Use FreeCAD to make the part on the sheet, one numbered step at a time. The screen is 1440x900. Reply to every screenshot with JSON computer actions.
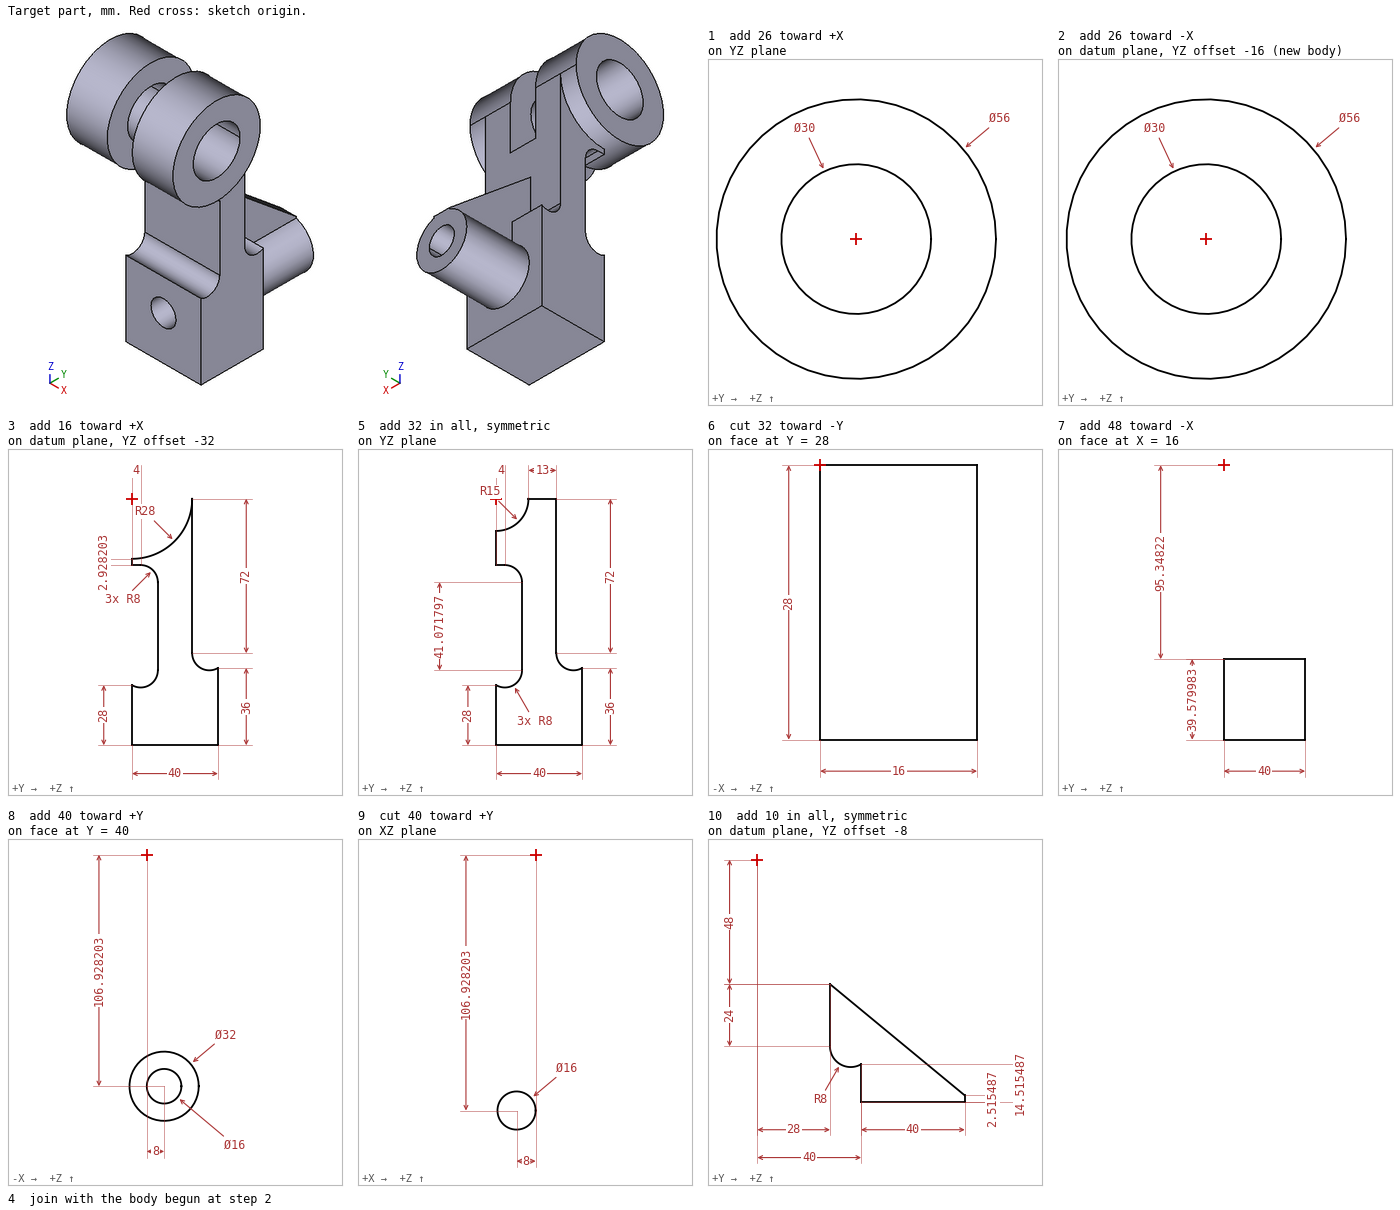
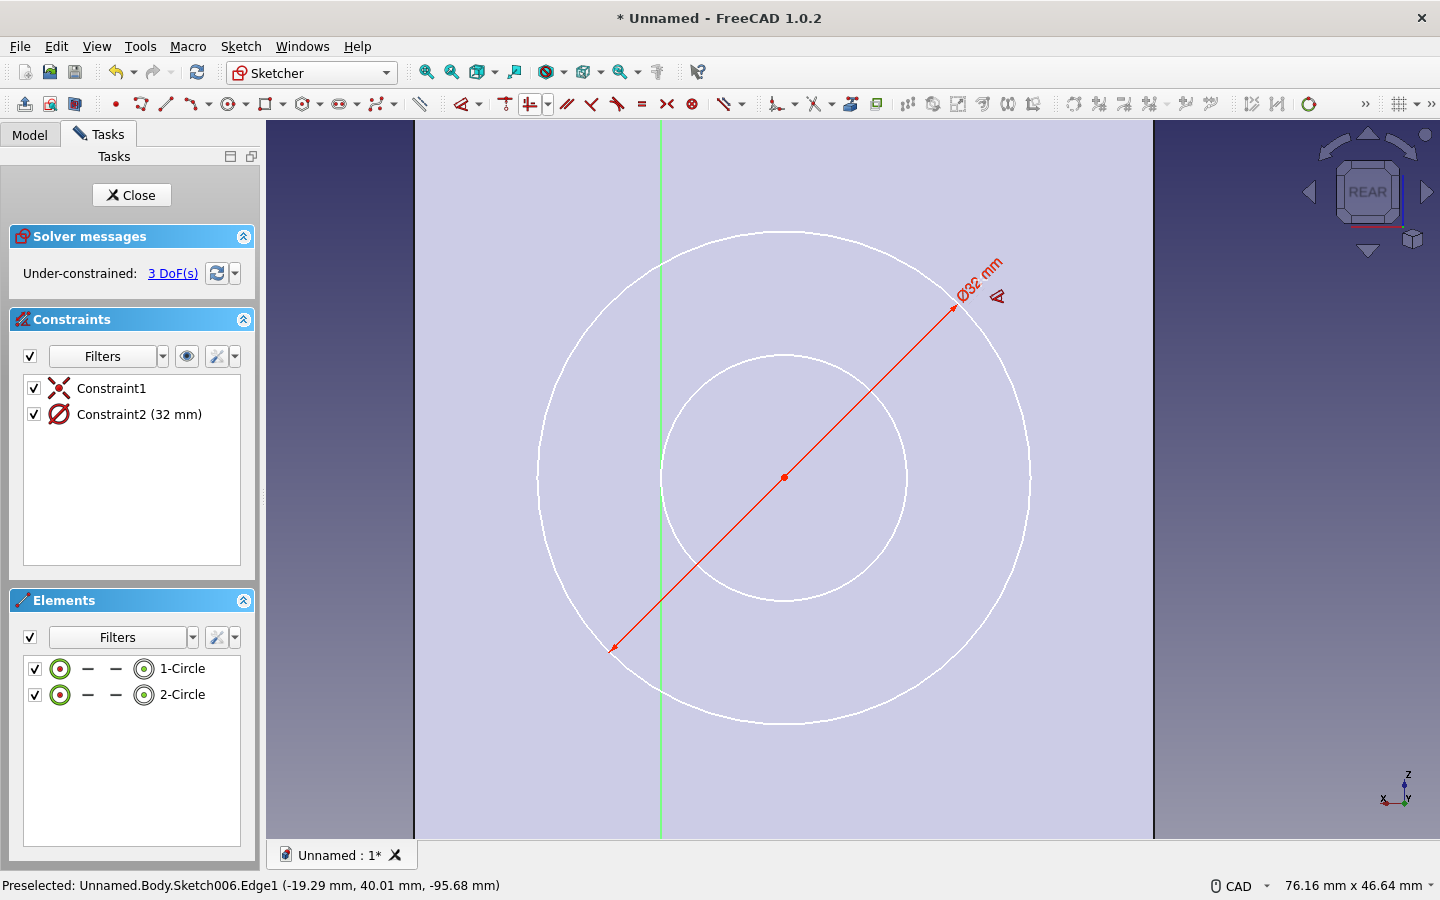
{"action": "left_click", "coordinate": [871, 391]}
{"action": "left_click", "coordinate": [894, 368]}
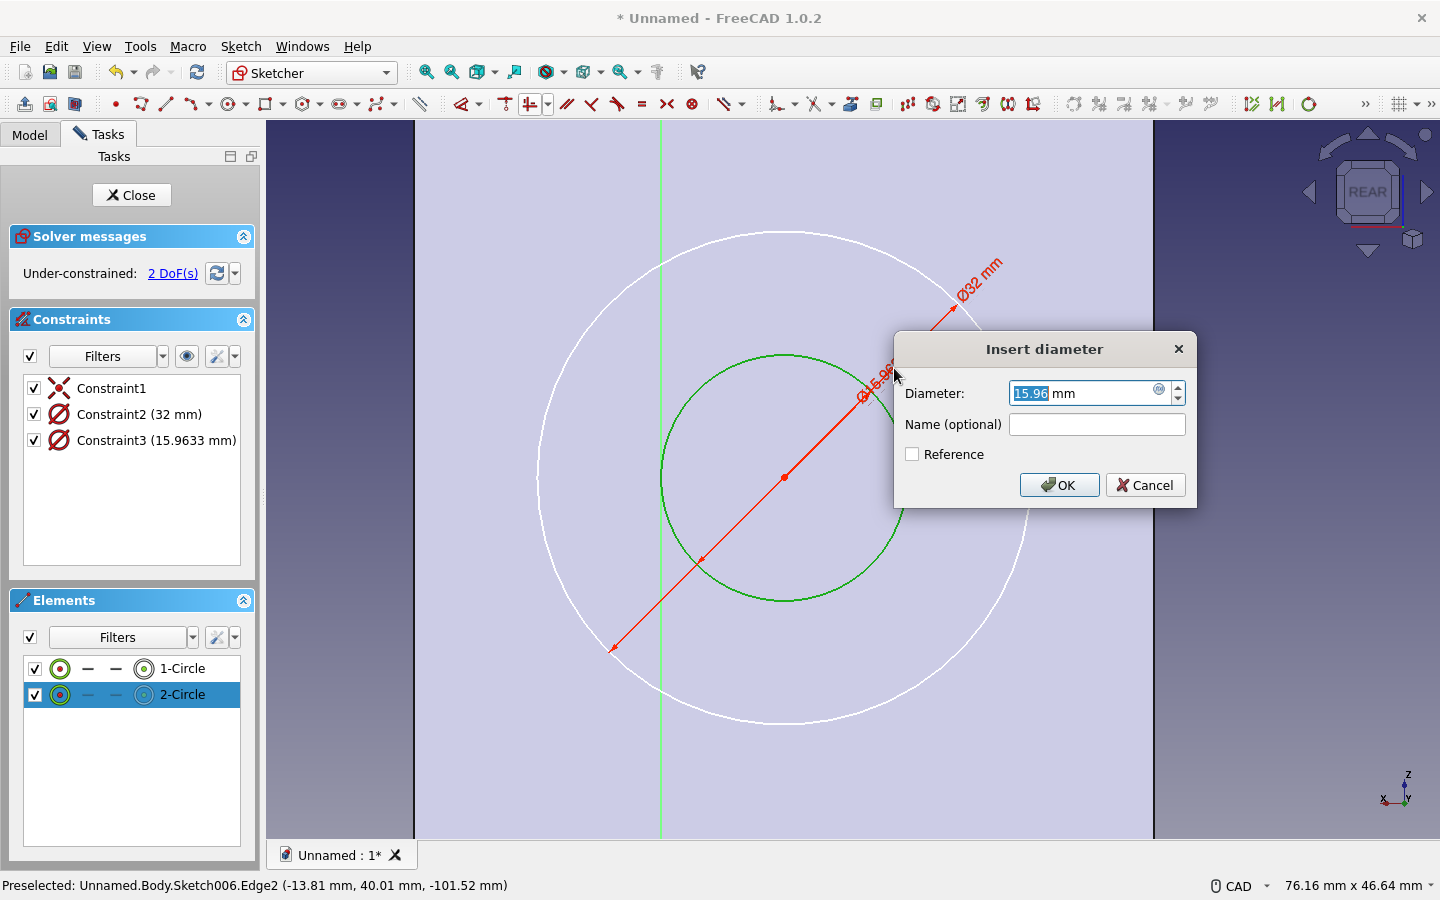
{"action": "type", "text": "16"}
{"action": "key", "text": "Return"}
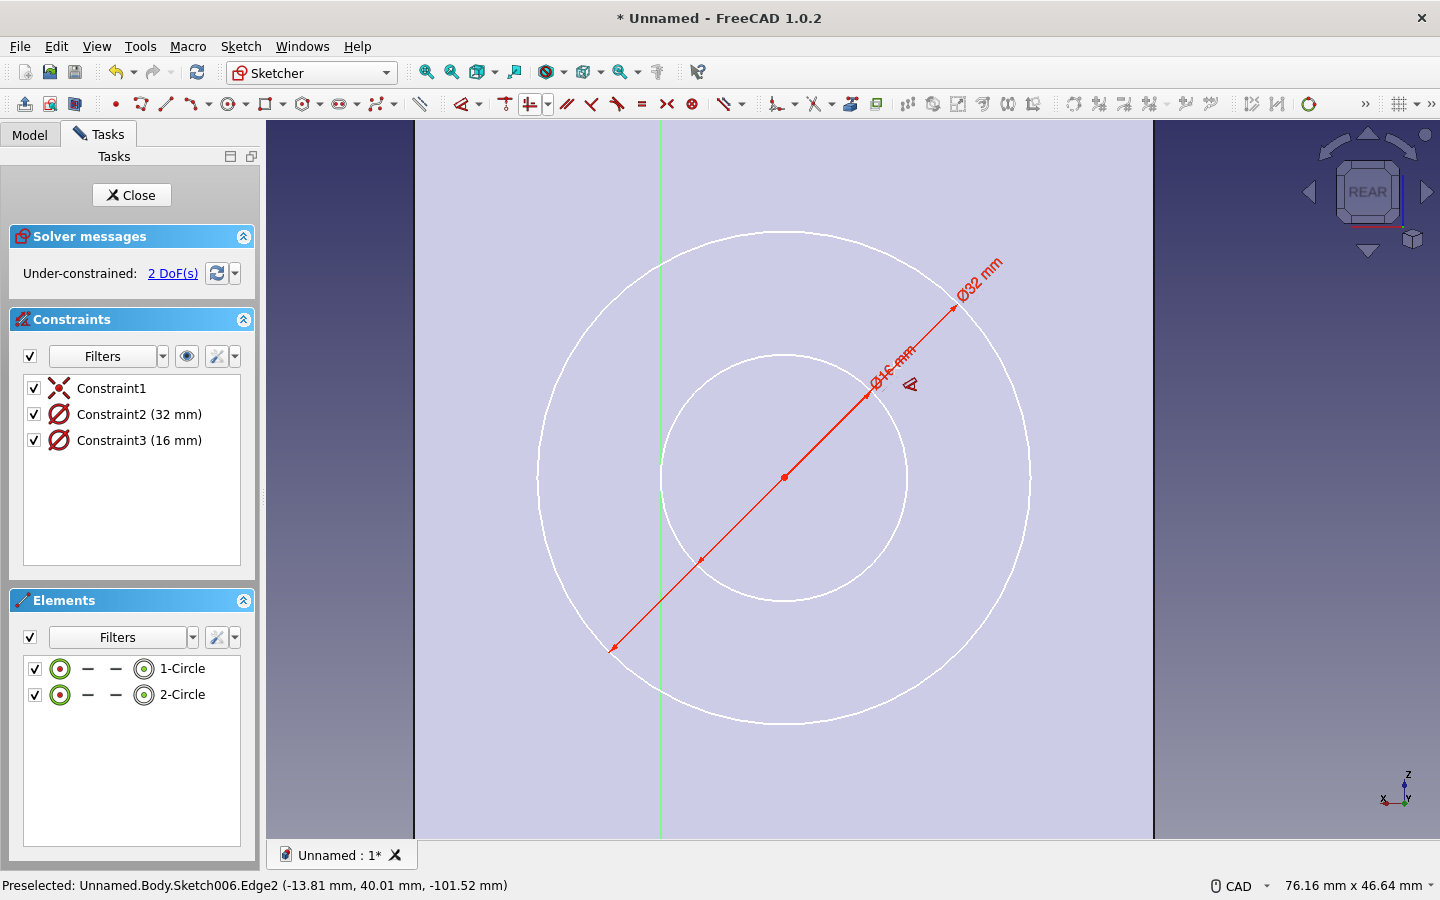
{"action": "left_click", "coordinate": [784, 478]}
{"action": "left_click", "coordinate": [722, 512]}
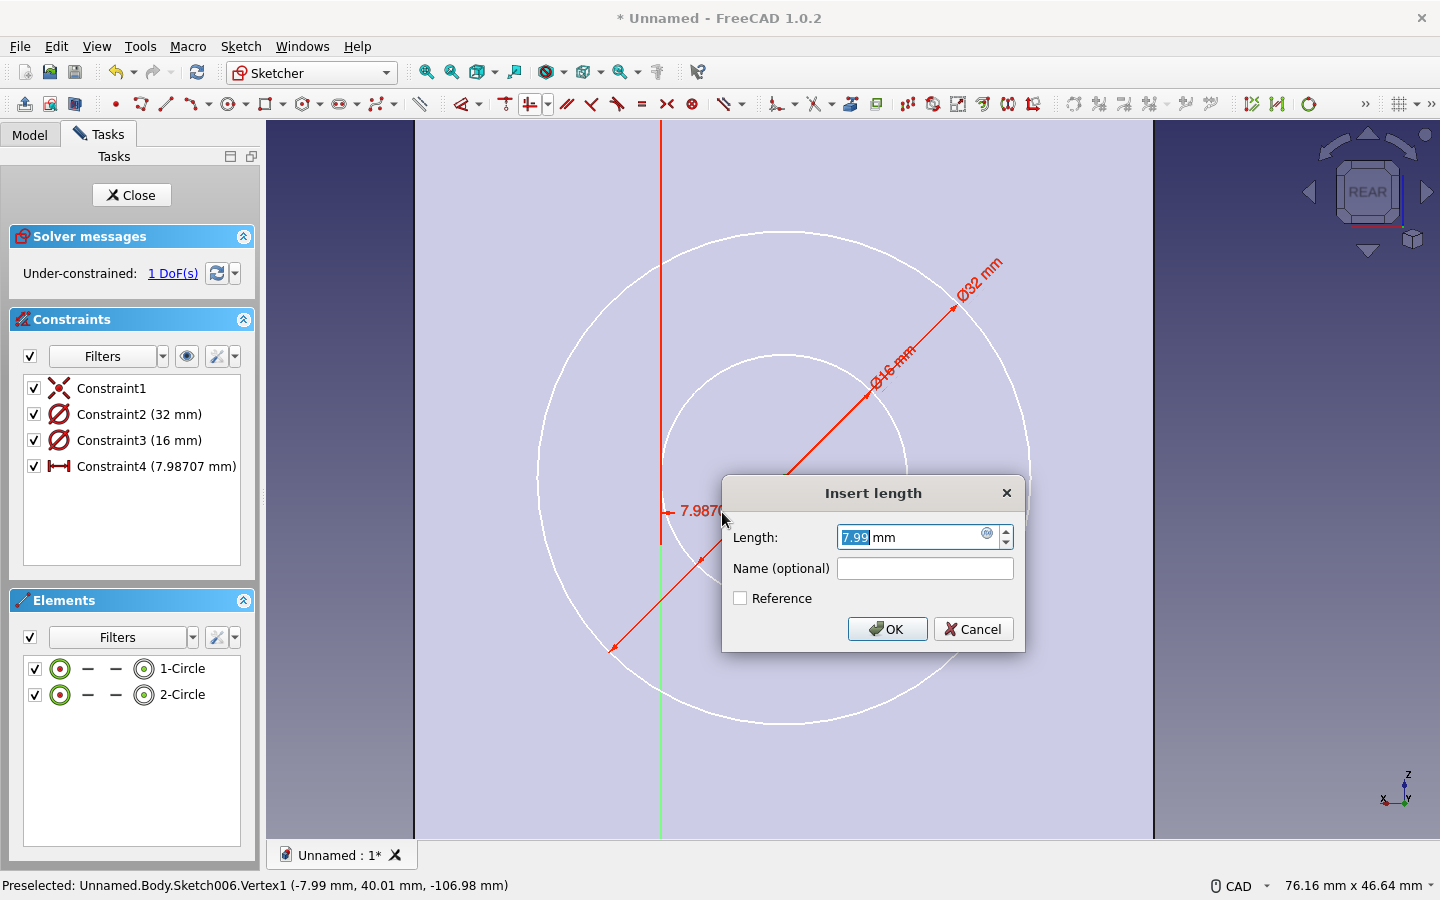
{"action": "type", "text": "8"}
{"action": "key", "text": "Return"}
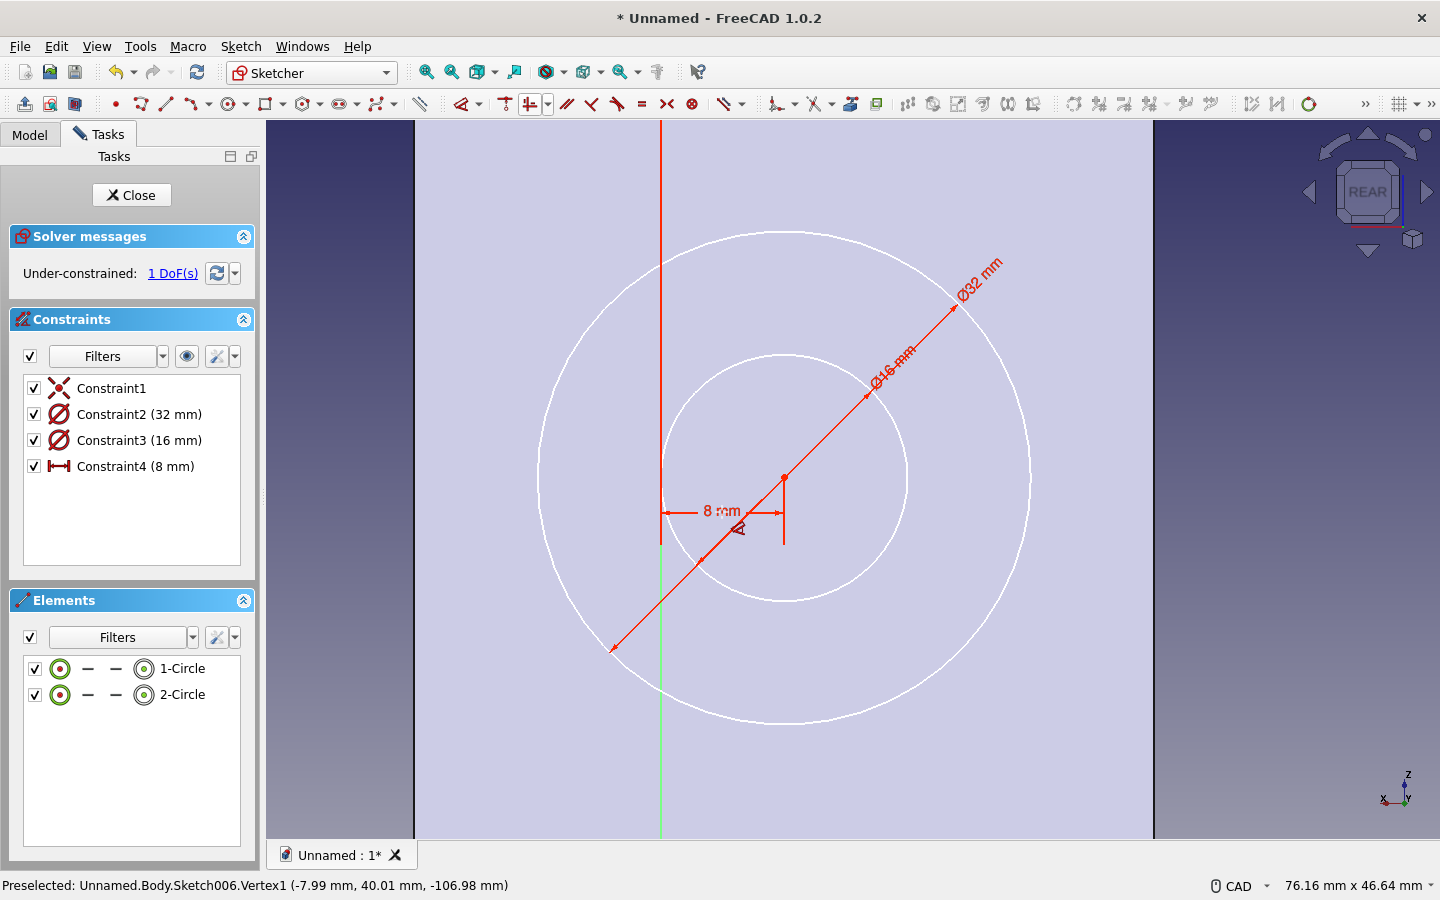
{"action": "left_click", "coordinate": [784, 478]}
{"action": "left_click", "coordinate": [627, 313]}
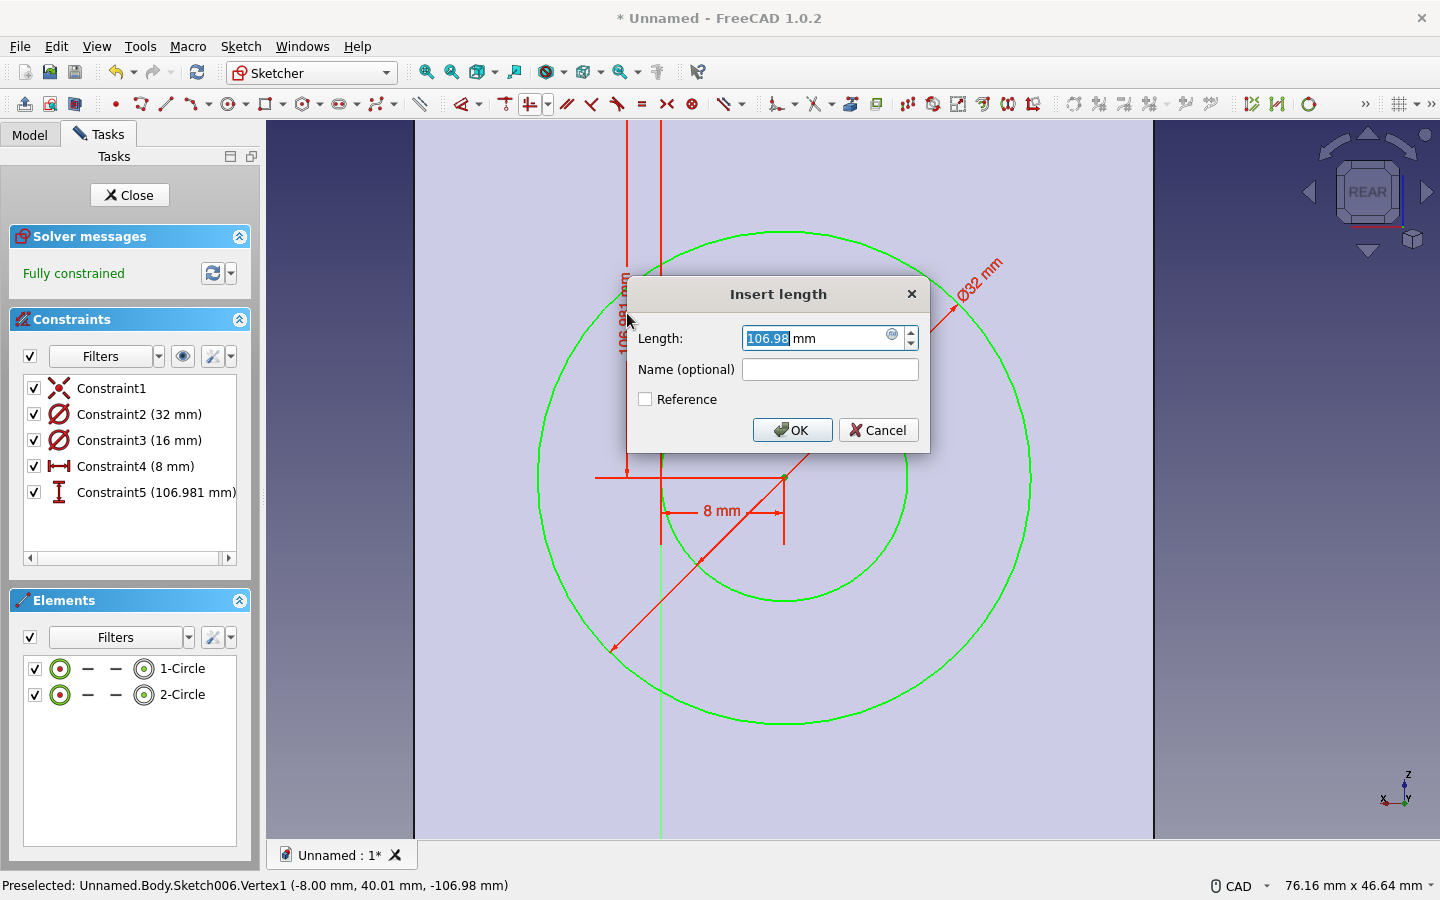
{"action": "type", "text": "106.928203"}
{"action": "key", "text": "Return"}
{"action": "key", "text": "Escape"}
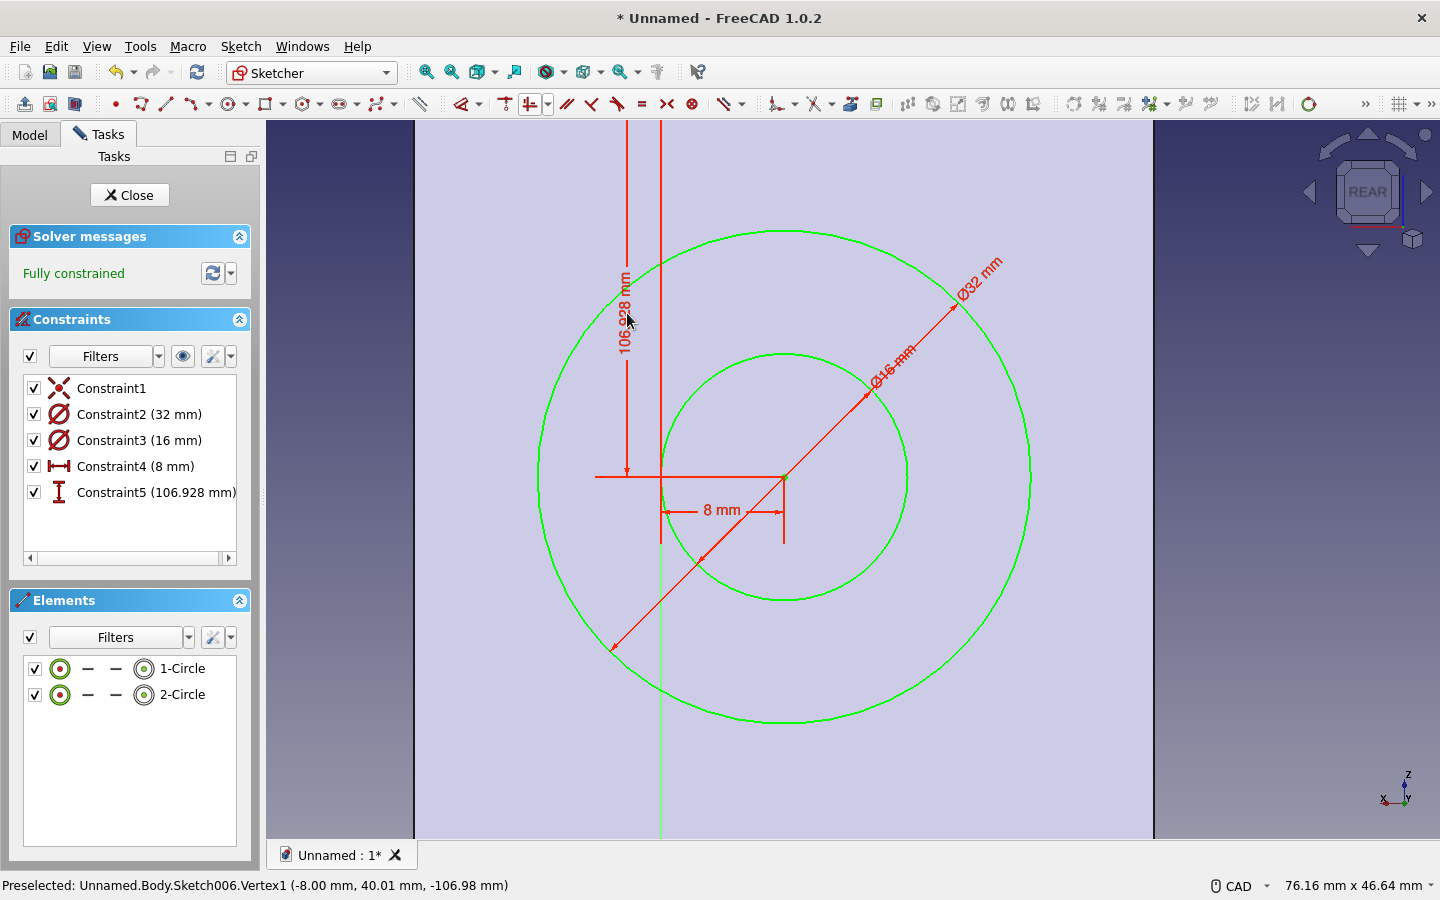
{"action": "left_click", "coordinate": [130, 195]}